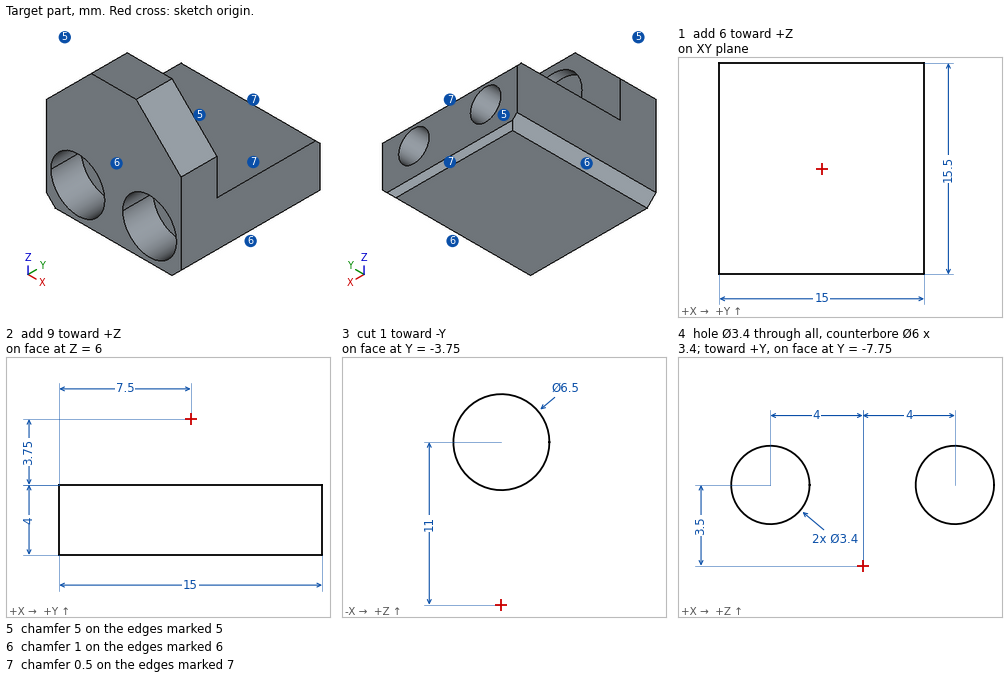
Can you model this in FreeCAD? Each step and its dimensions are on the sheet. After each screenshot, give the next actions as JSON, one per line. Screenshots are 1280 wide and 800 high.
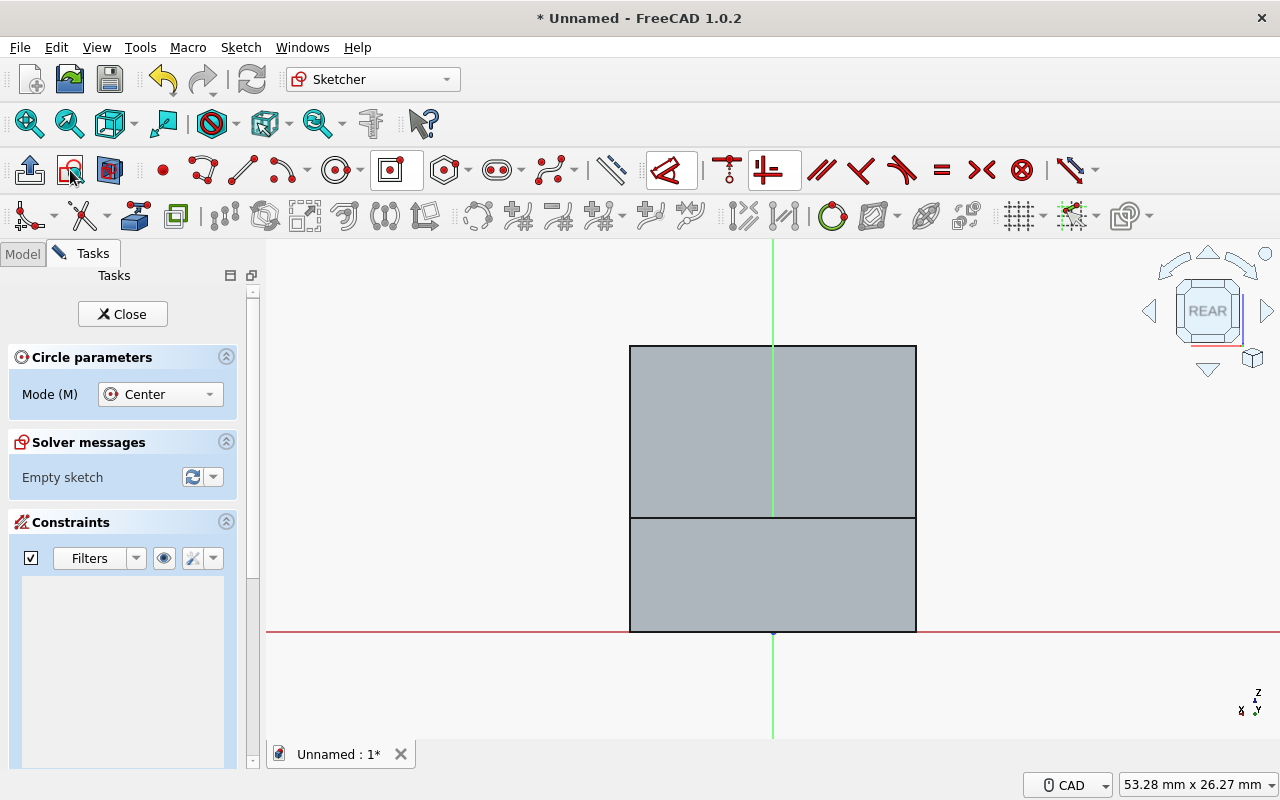
{"action": "left_click", "coordinate": [773, 422]}
{"action": "left_click", "coordinate": [817, 379]}
{"action": "key", "text": "Escape"}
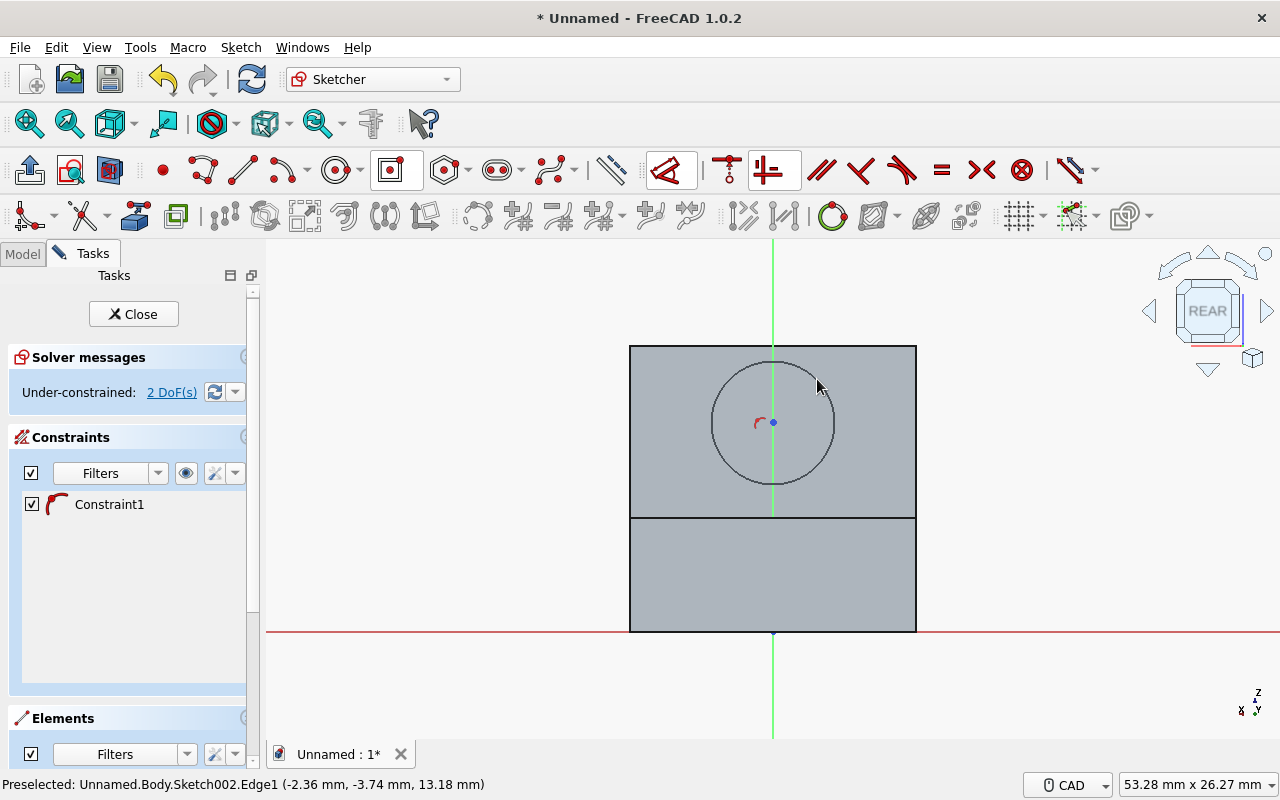
{"action": "key", "text": "d"}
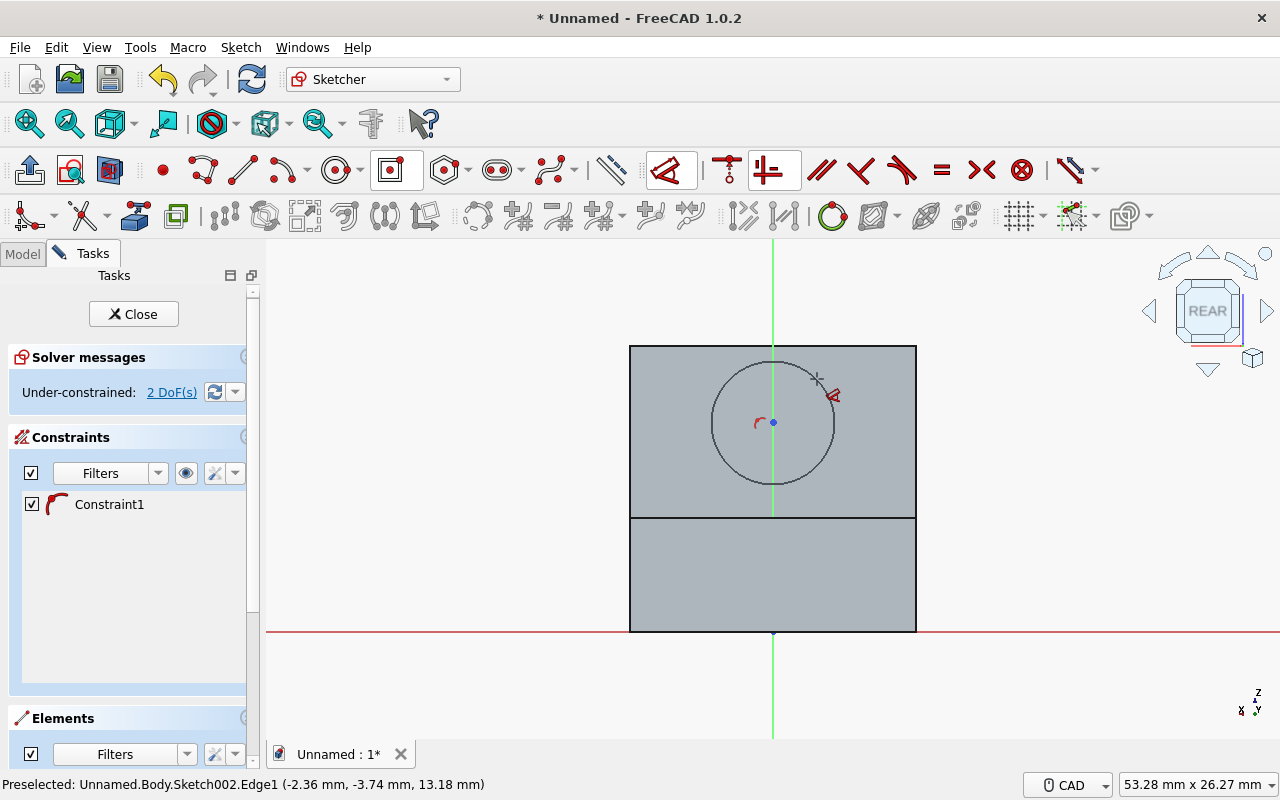
{"action": "left_click", "coordinate": [816, 379]}
{"action": "left_click", "coordinate": [838, 356]}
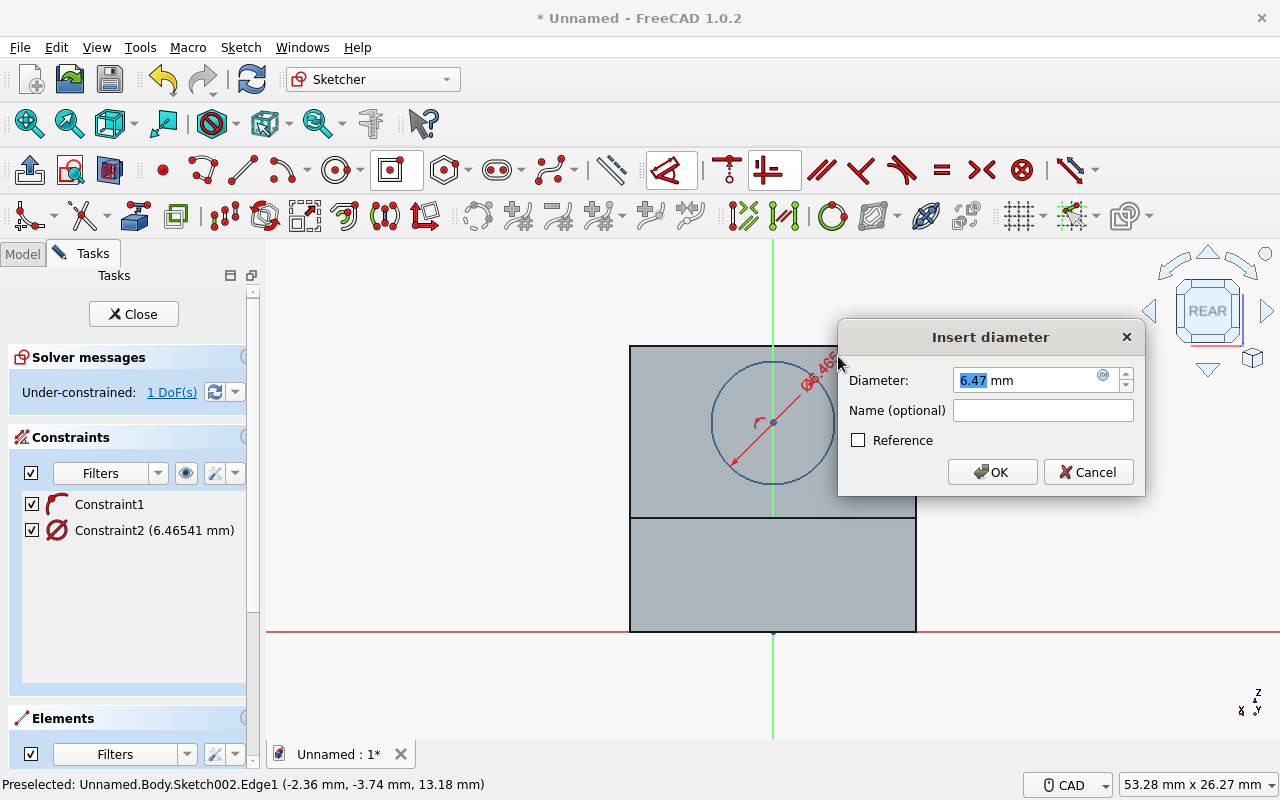
{"action": "type", "text": "6.5"}
{"action": "key", "text": "Return"}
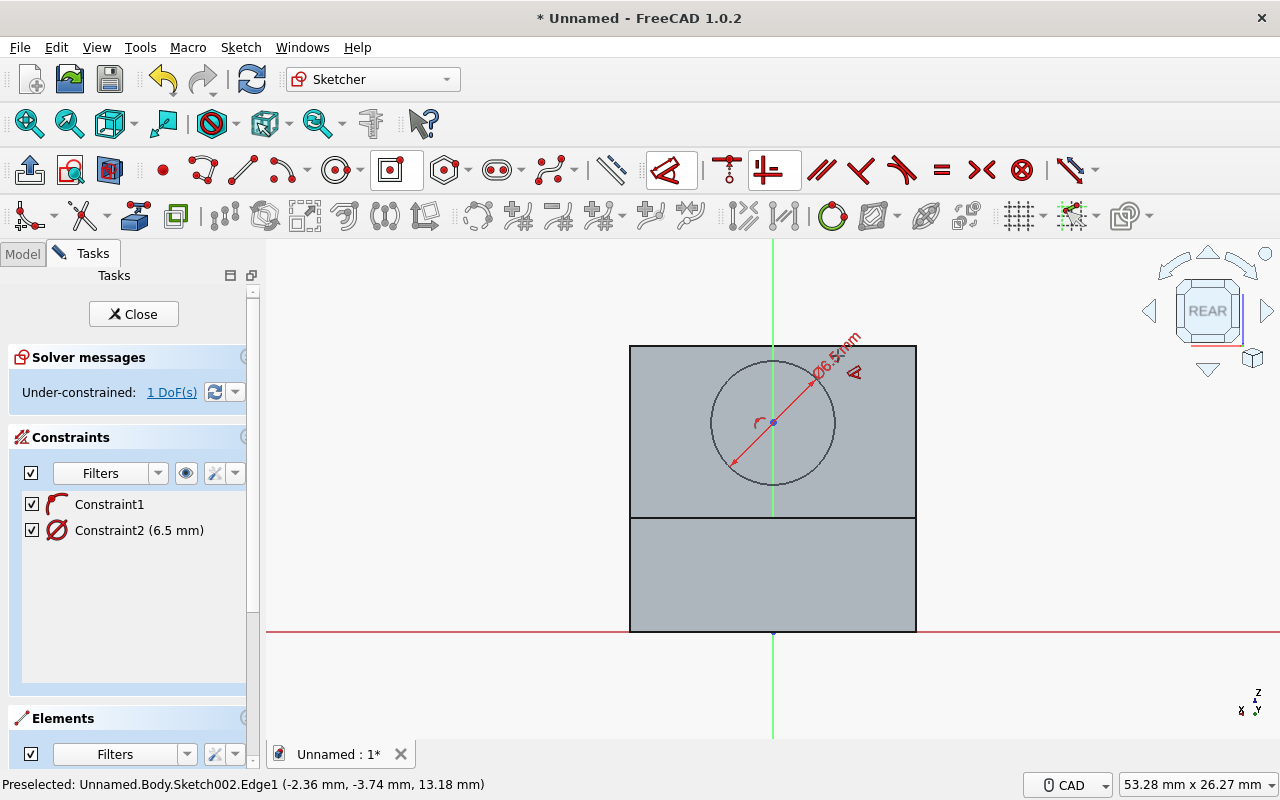
{"action": "left_click", "coordinate": [773, 423]}
{"action": "left_click", "coordinate": [807, 527]}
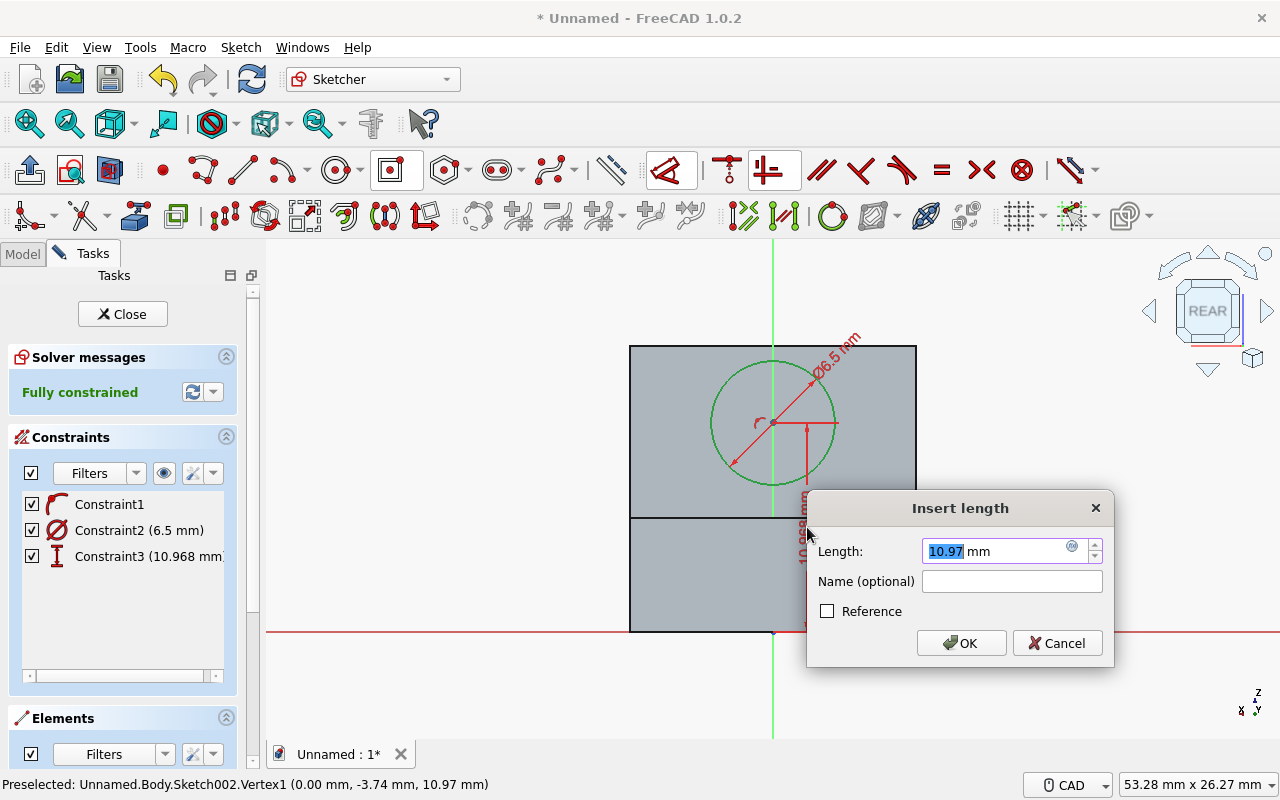
{"action": "type", "text": "11"}
{"action": "key", "text": "Return"}
{"action": "key", "text": "Escape"}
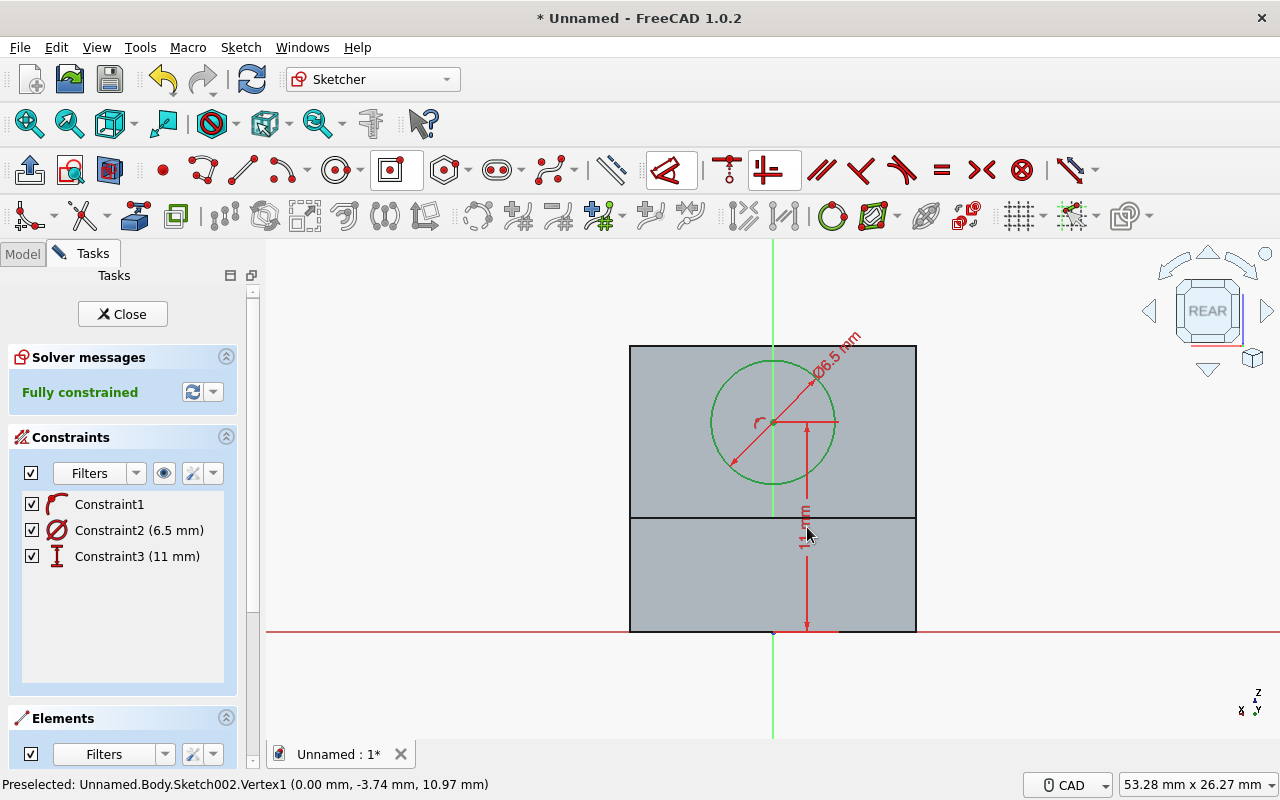
{"action": "left_click", "coordinate": [123, 314]}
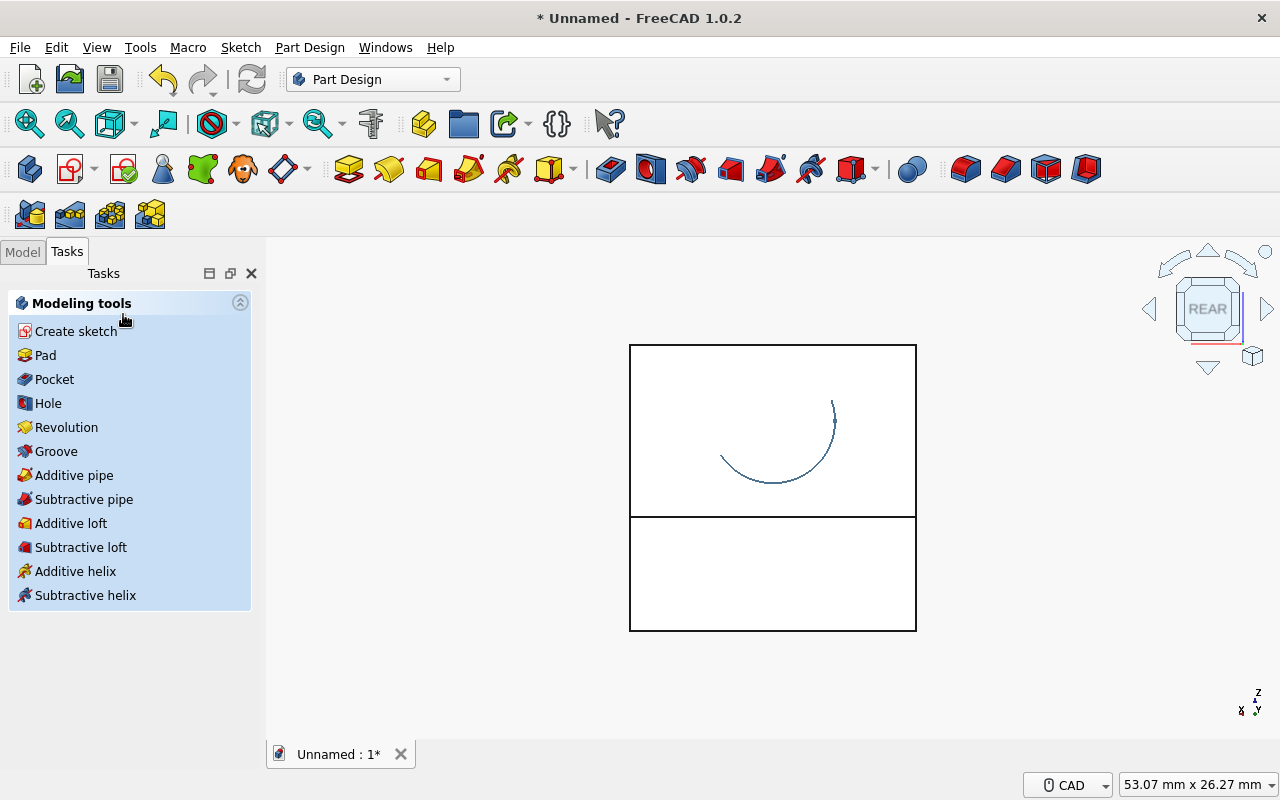
{"action": "left_click", "coordinate": [612, 170]}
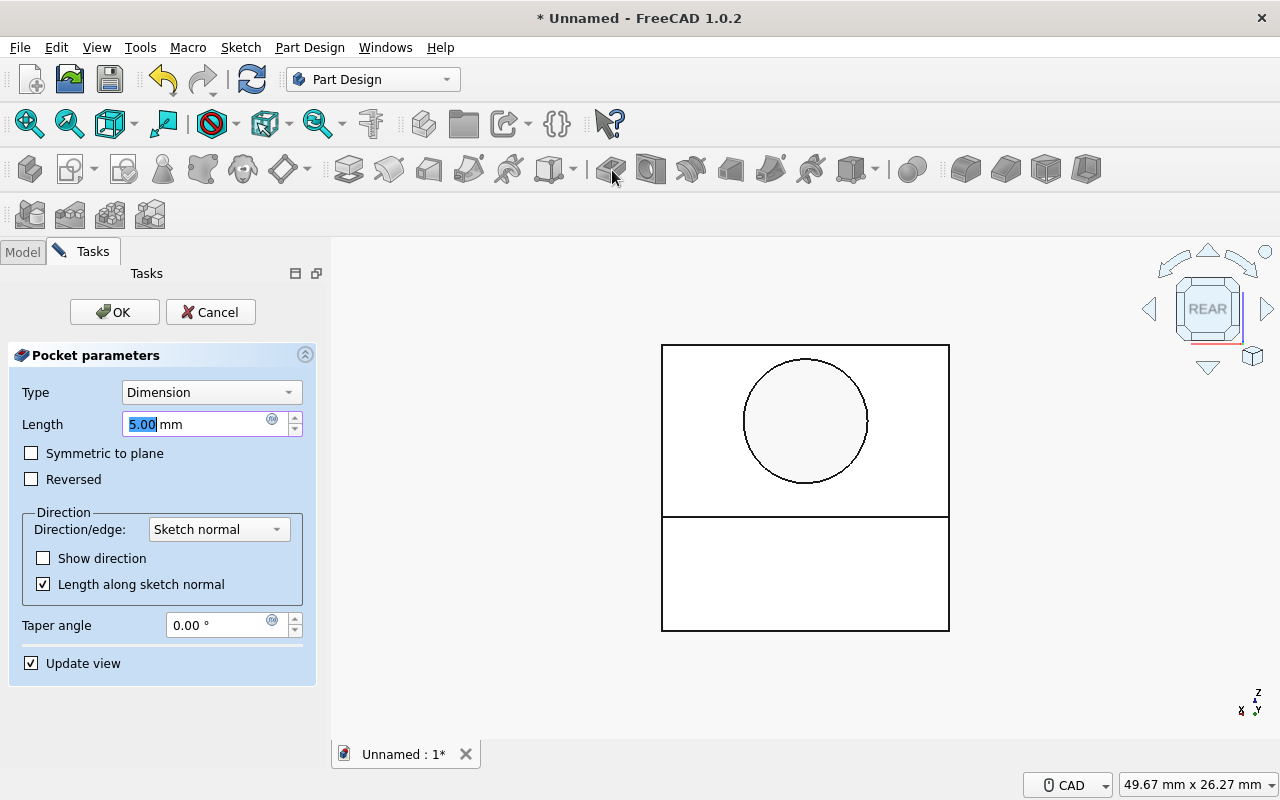
{"action": "type", "text": "1"}
{"action": "key", "text": "Tab"}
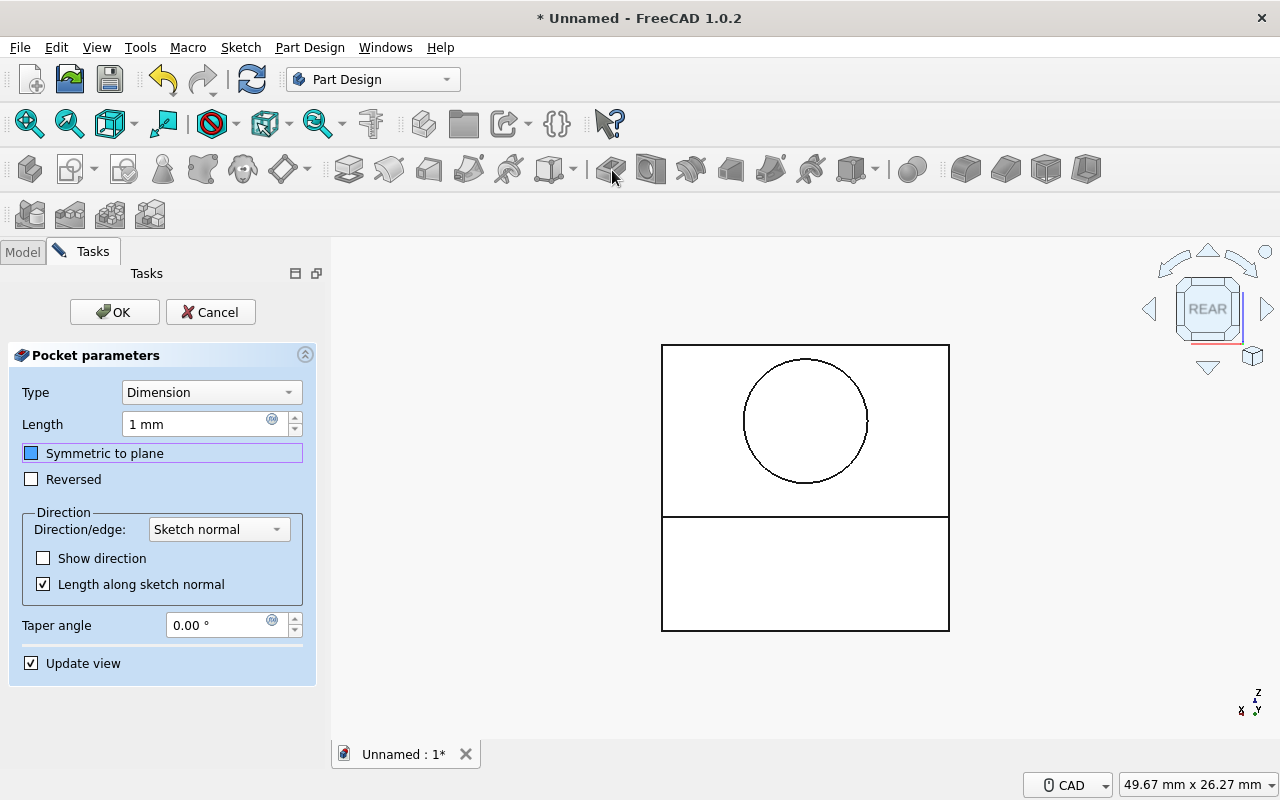
{"action": "left_click", "coordinate": [115, 312]}